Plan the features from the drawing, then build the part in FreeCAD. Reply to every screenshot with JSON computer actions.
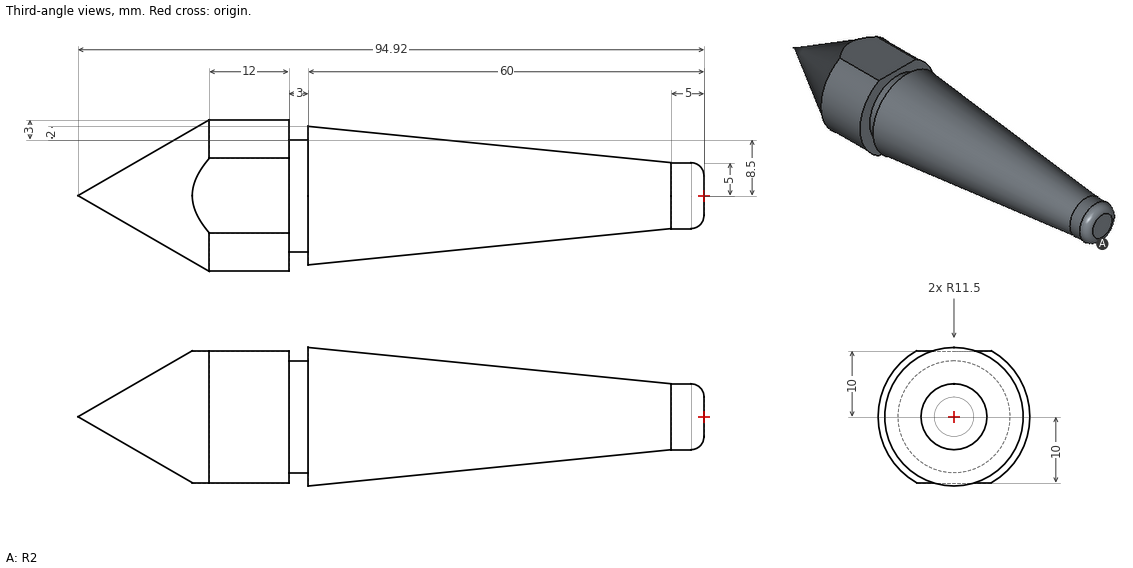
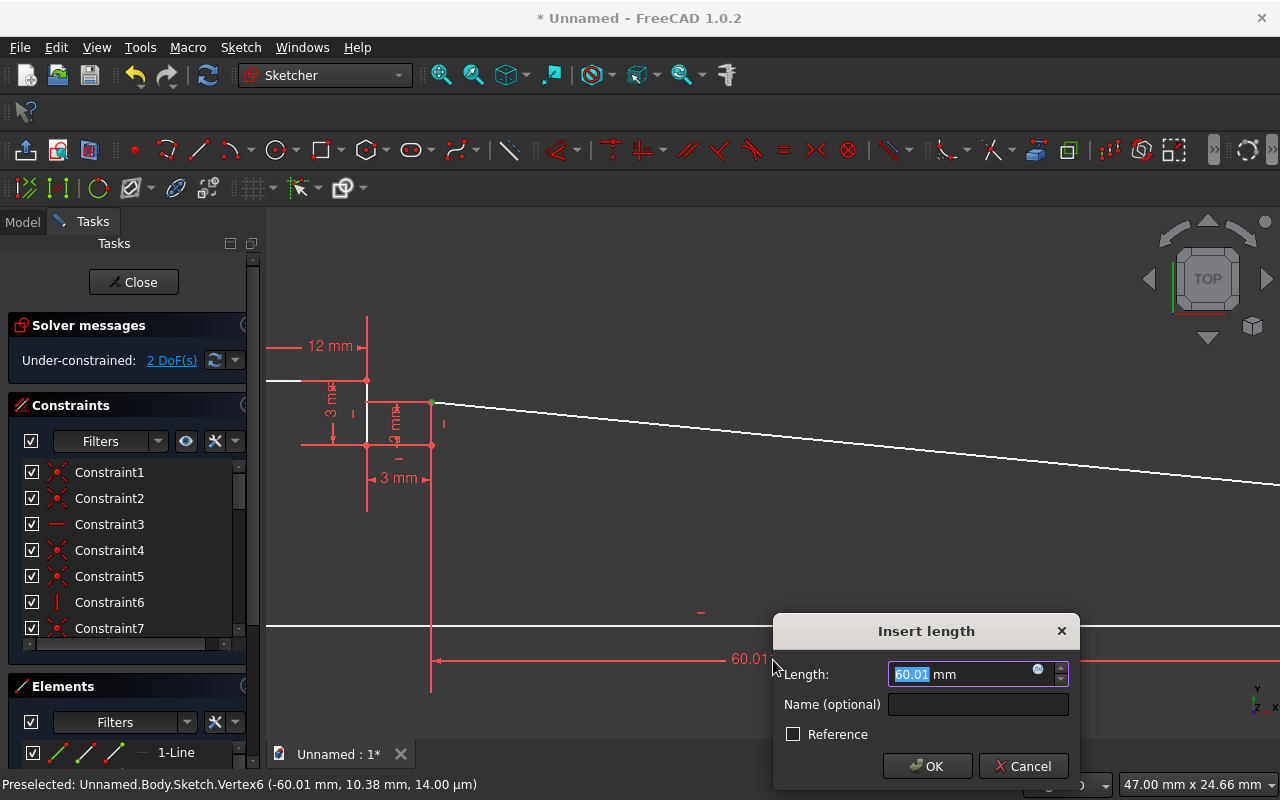
{"action": "type", "text": "60"}
{"action": "key", "text": "Return"}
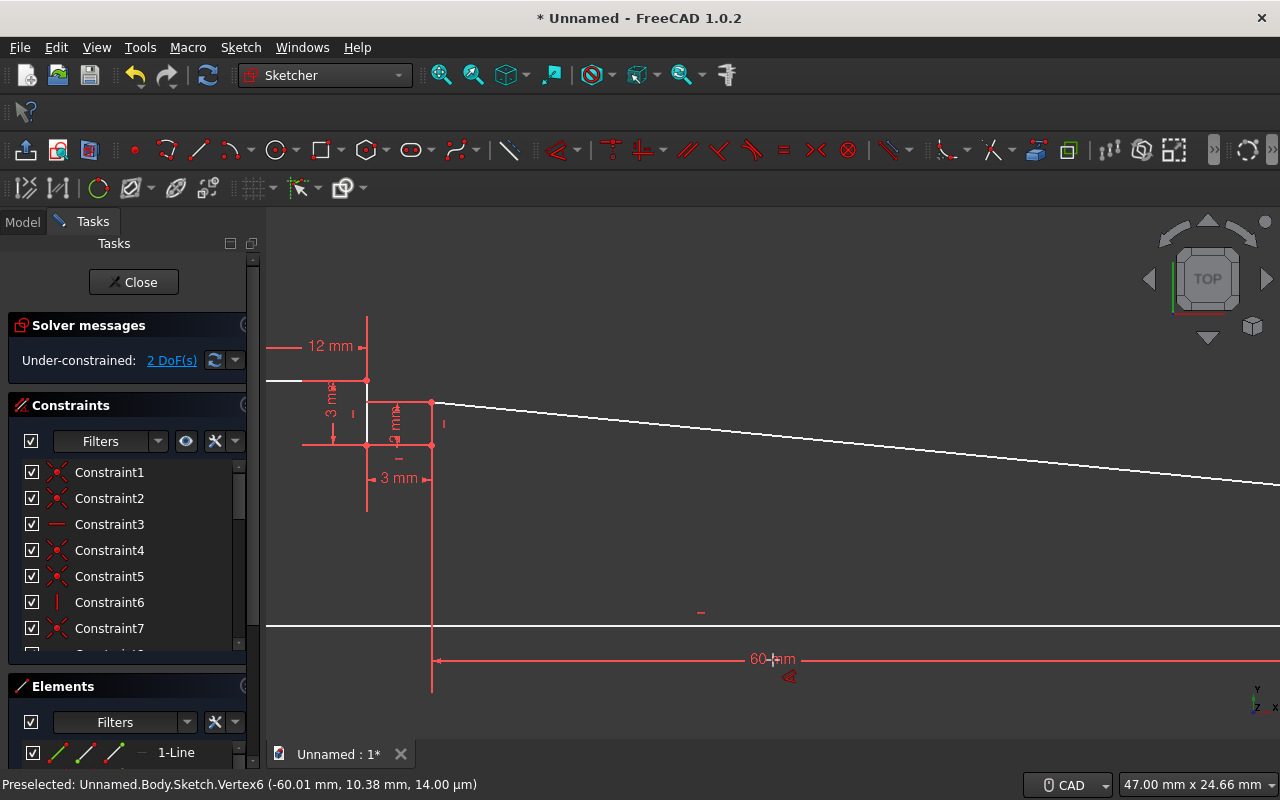
{"action": "left_click", "coordinate": [432, 445]}
{"action": "left_click", "coordinate": [398, 536]}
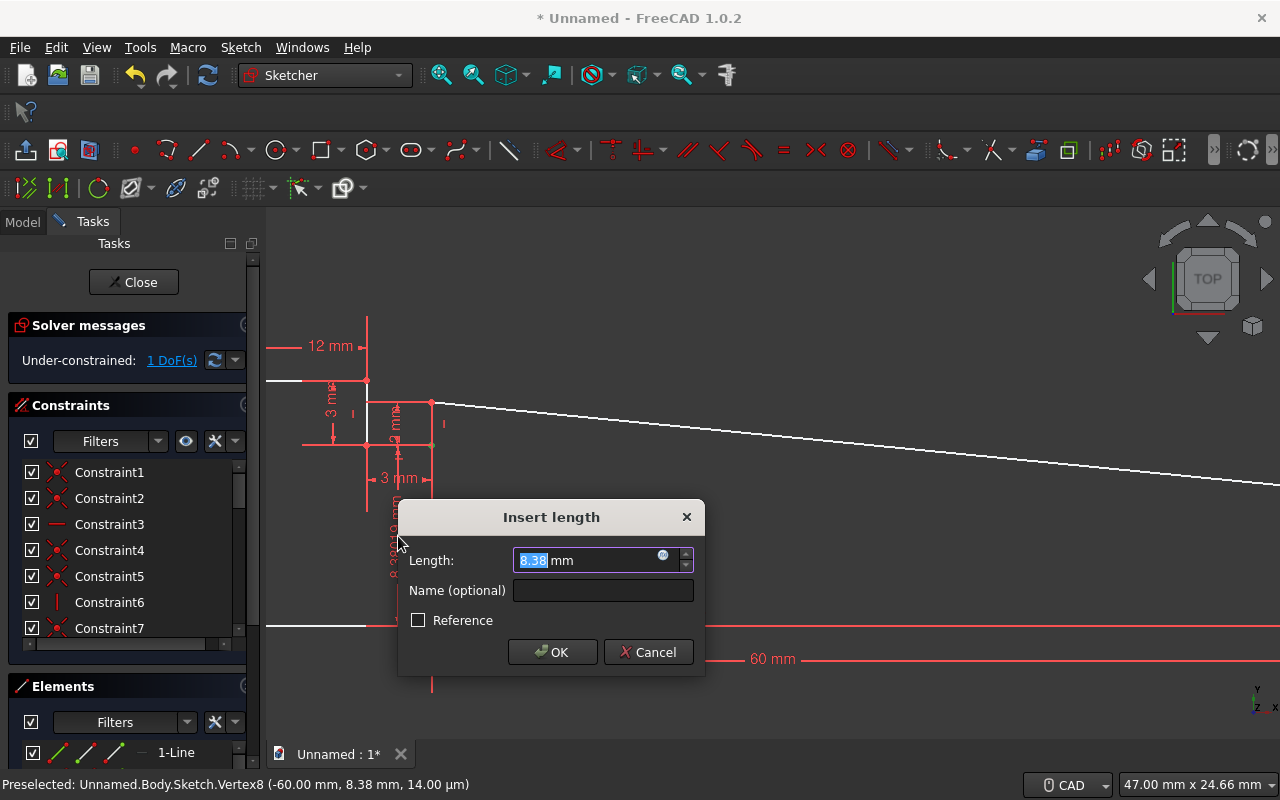
{"action": "type", "text": "8.5"}
{"action": "key", "text": "Return"}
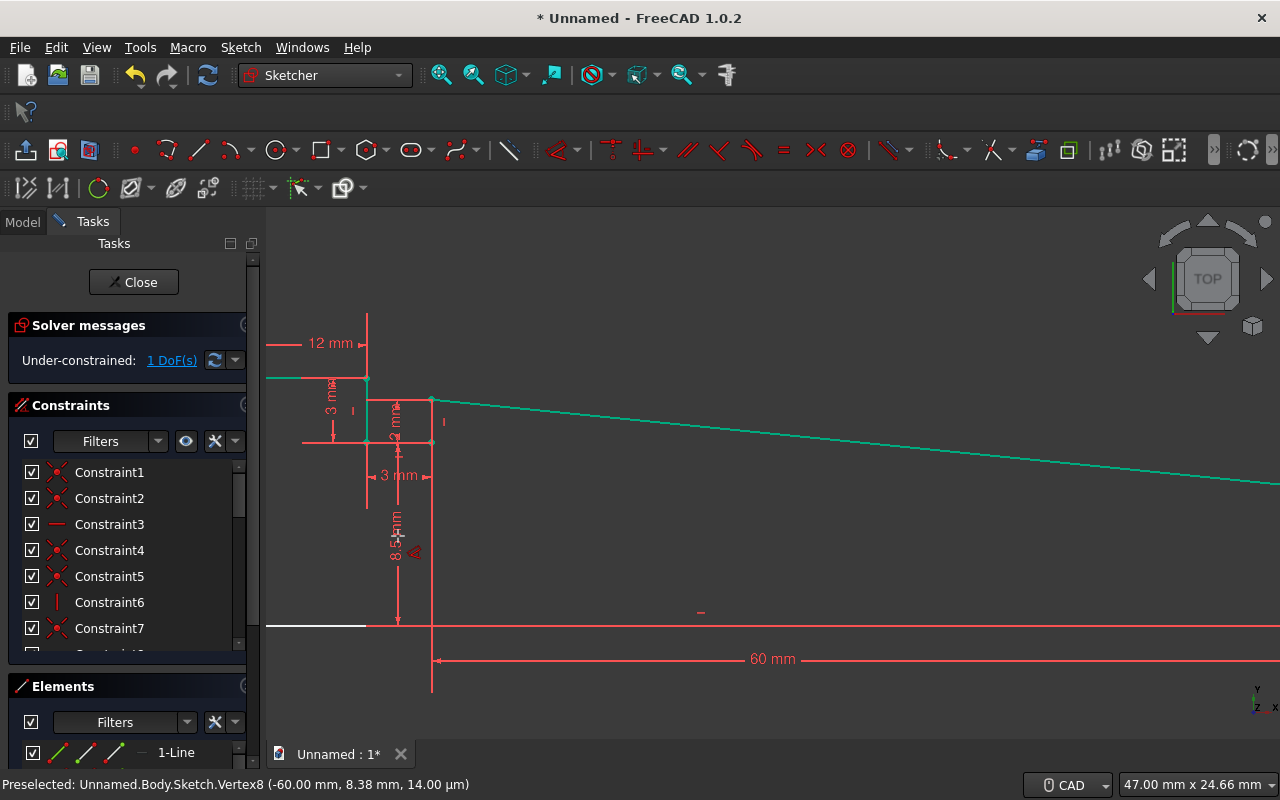
{"action": "left_click", "coordinate": [1112, 626]}
{"action": "left_click", "coordinate": [516, 660]}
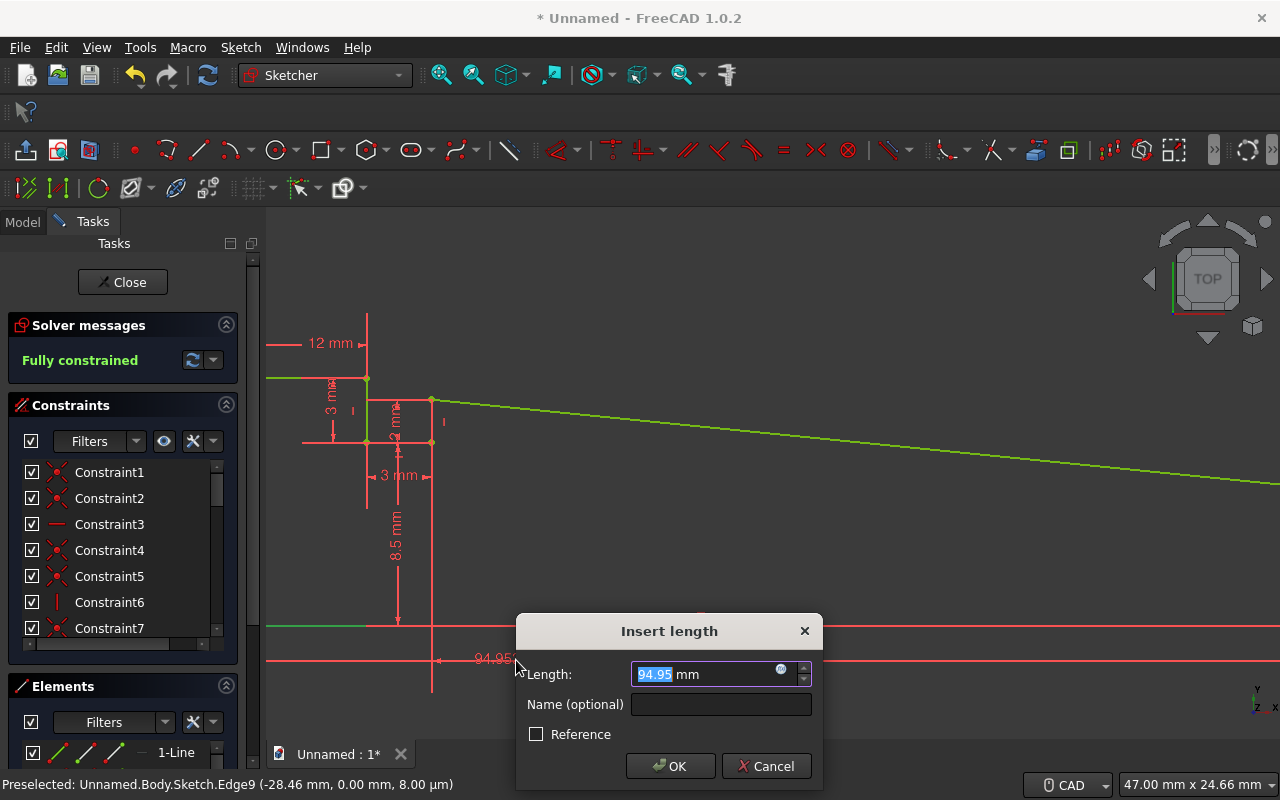
{"action": "type", "text": "94.92"}
{"action": "key", "text": "Return"}
{"action": "key", "text": "Escape"}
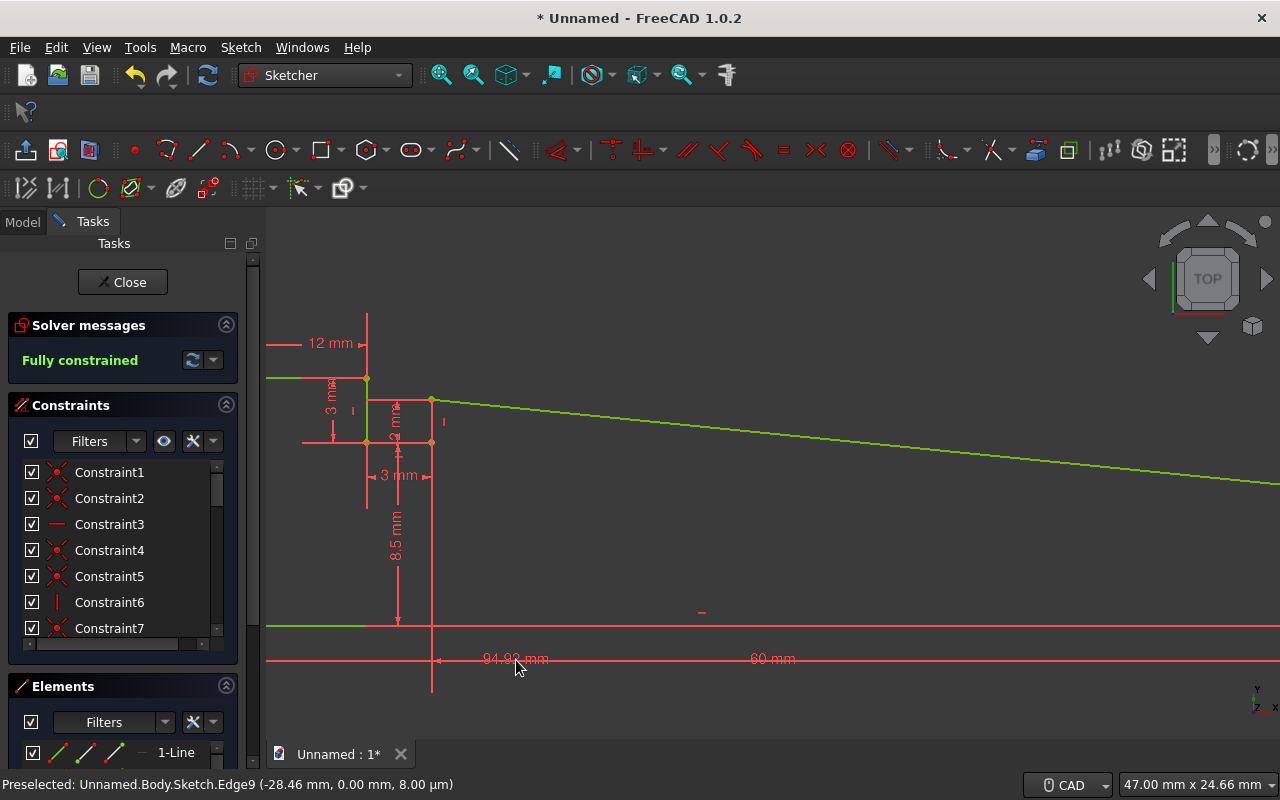
{"action": "left_click", "coordinate": [123, 282]}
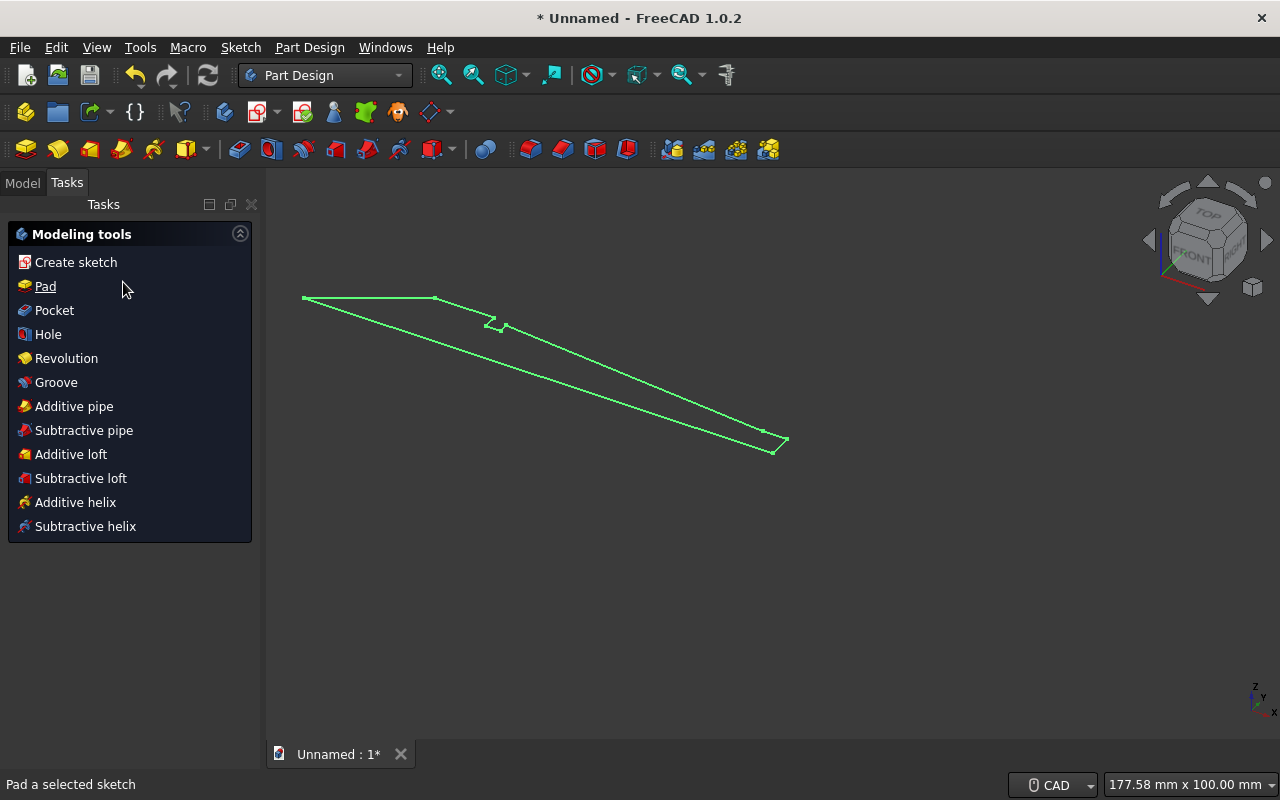
{"action": "left_click", "coordinate": [58, 150]}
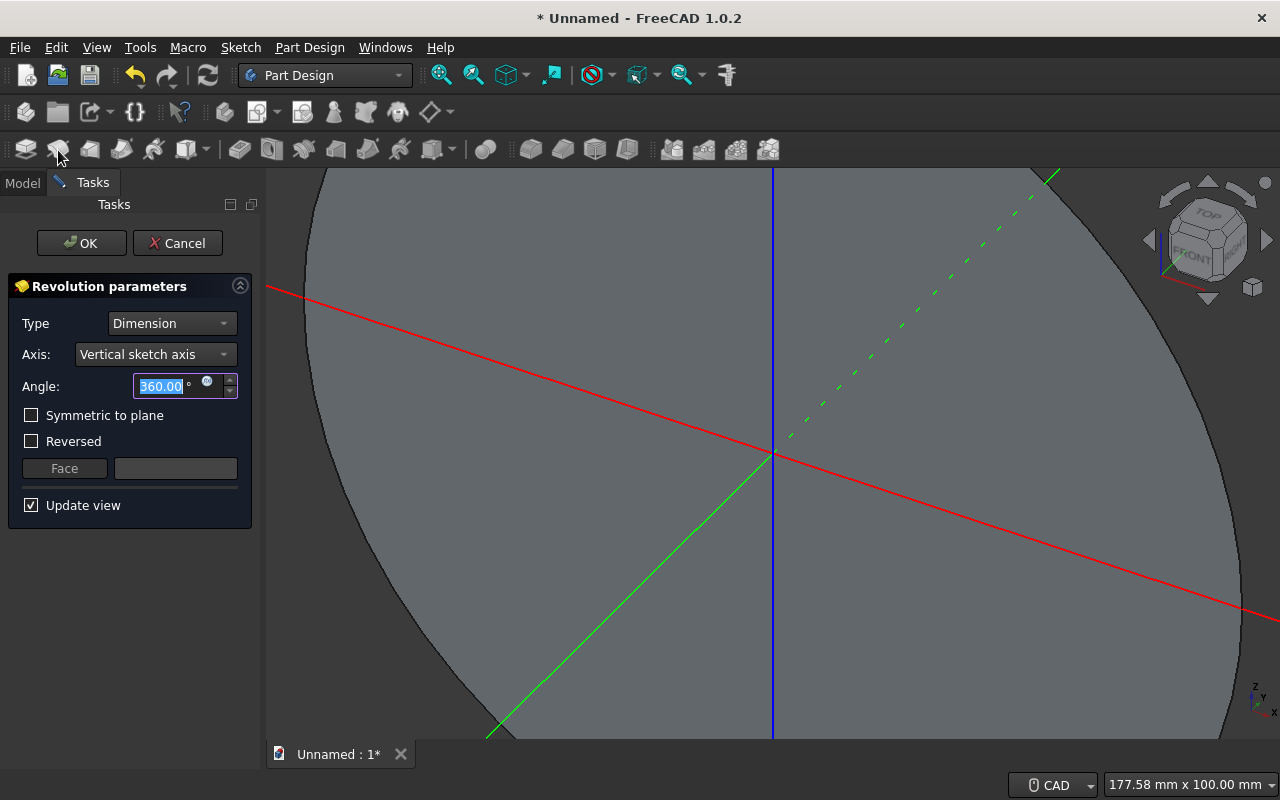
{"action": "left_click", "coordinate": [156, 354]}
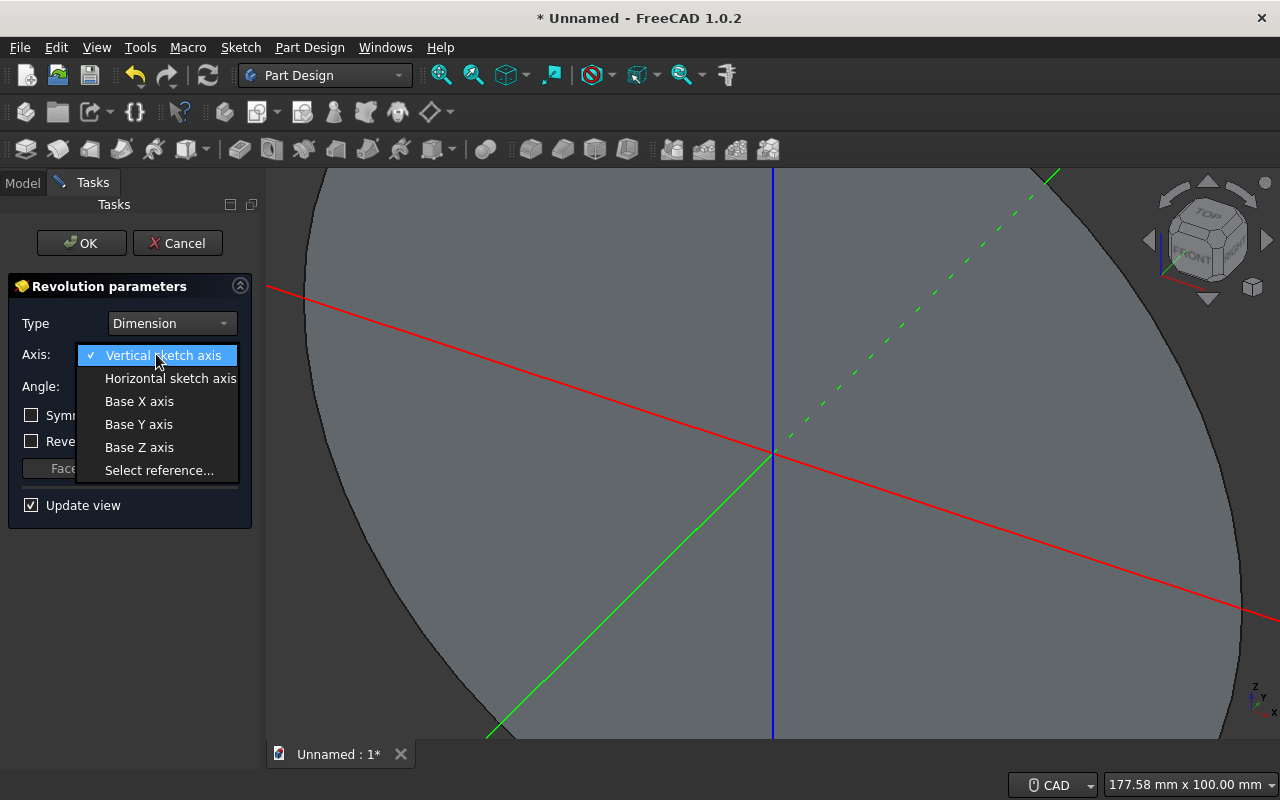
{"action": "left_click", "coordinate": [156, 378]}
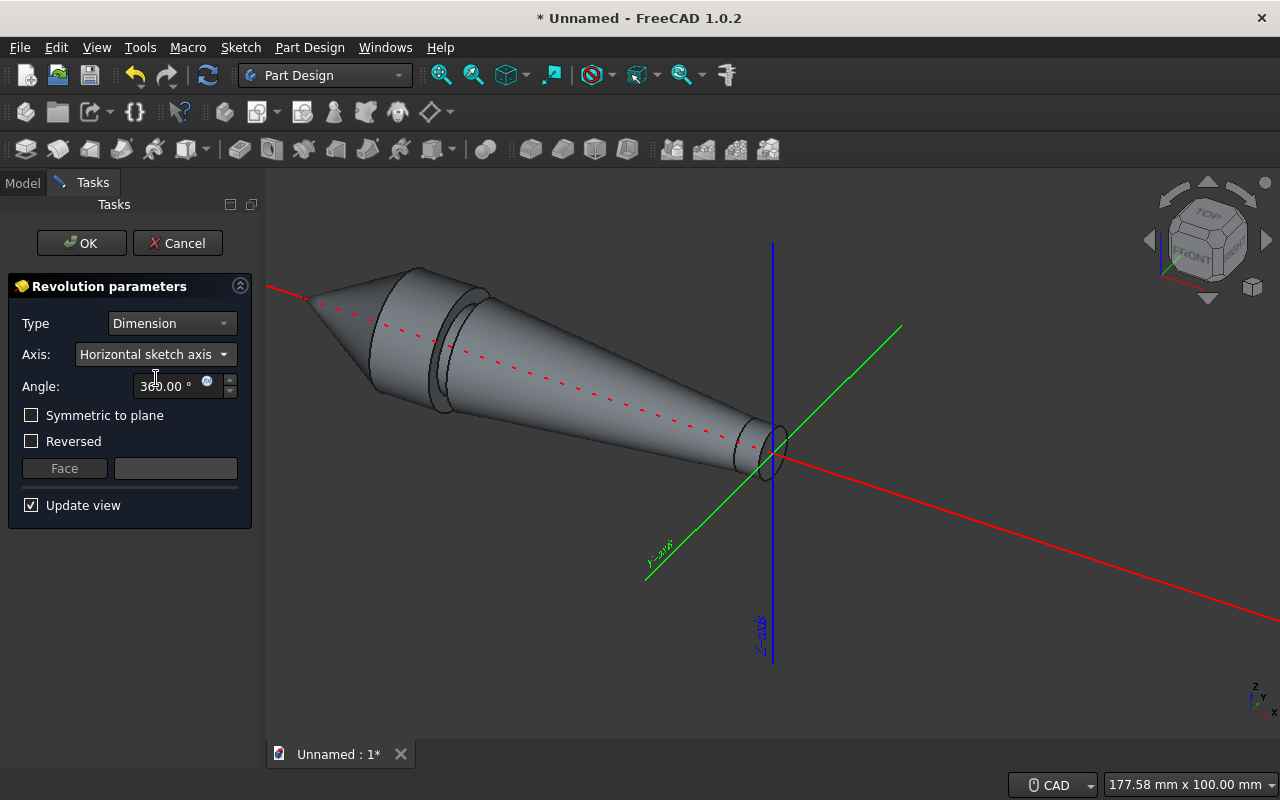
{"action": "left_click", "coordinate": [82, 243]}